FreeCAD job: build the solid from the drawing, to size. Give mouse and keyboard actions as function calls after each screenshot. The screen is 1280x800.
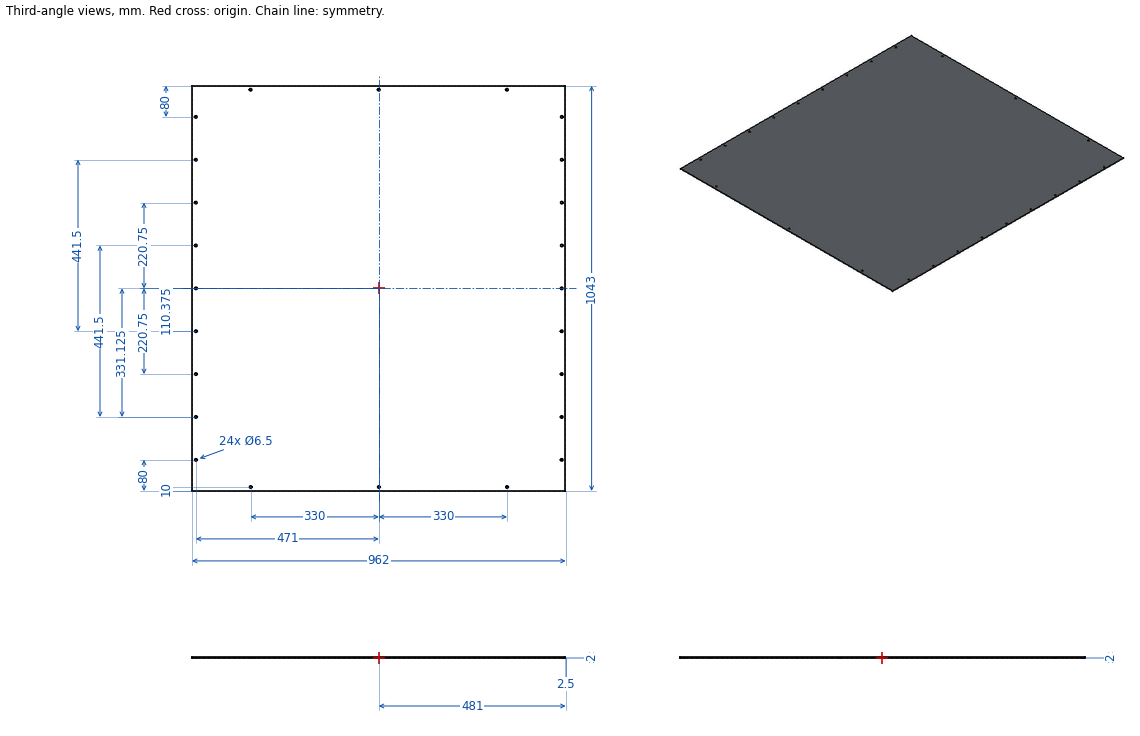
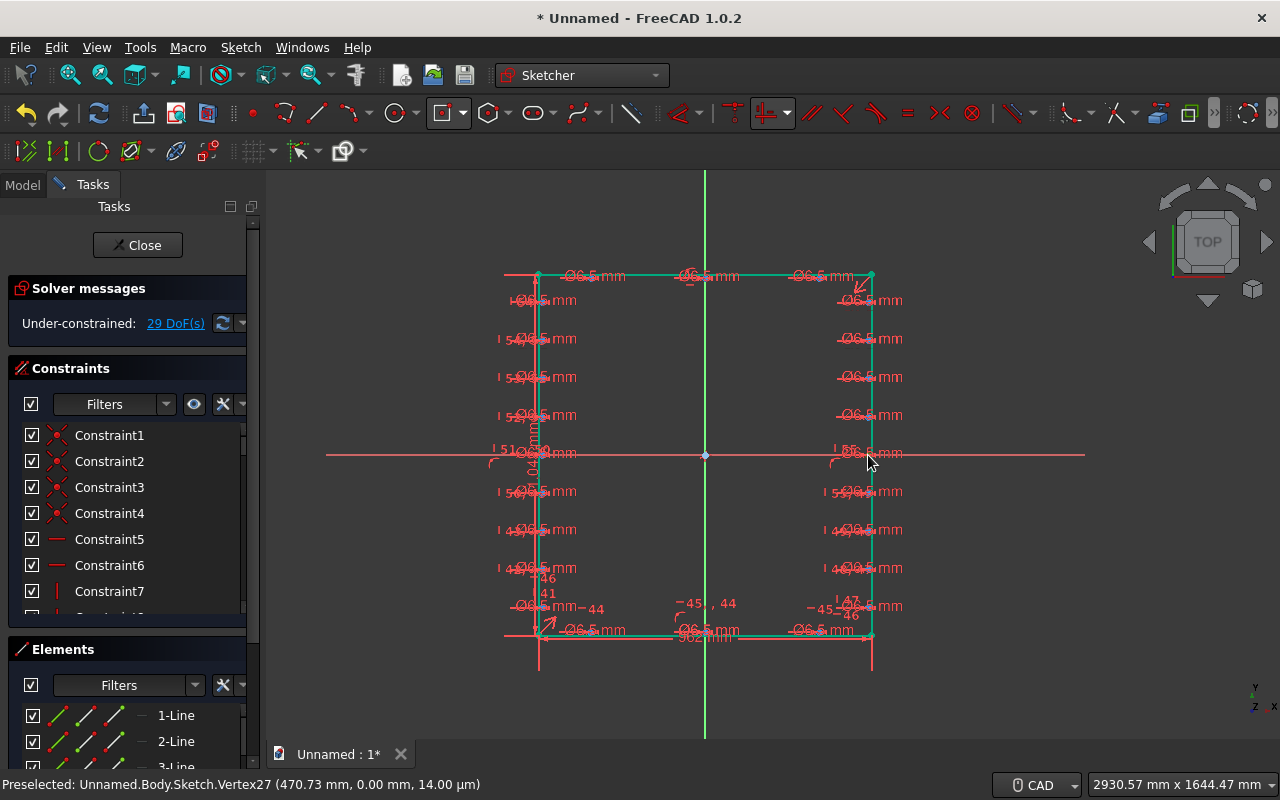
click(868, 417)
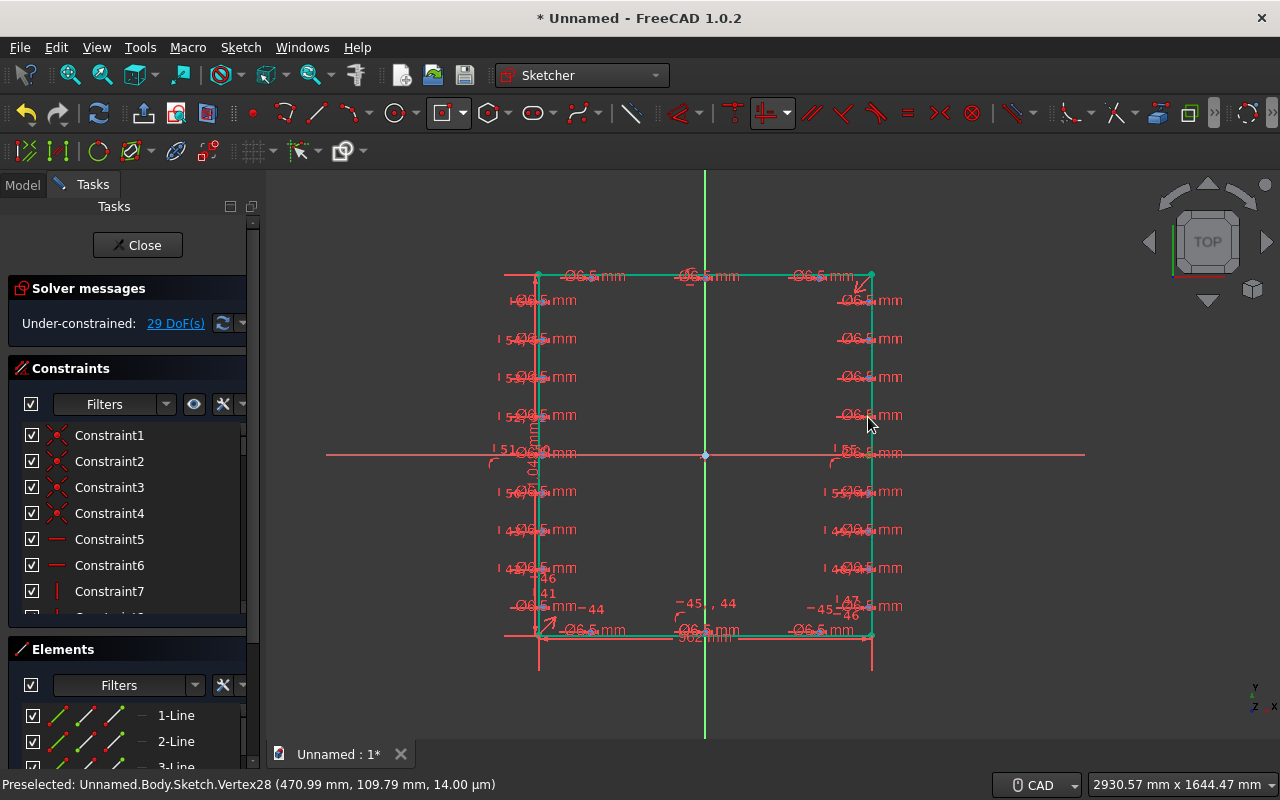
key(v)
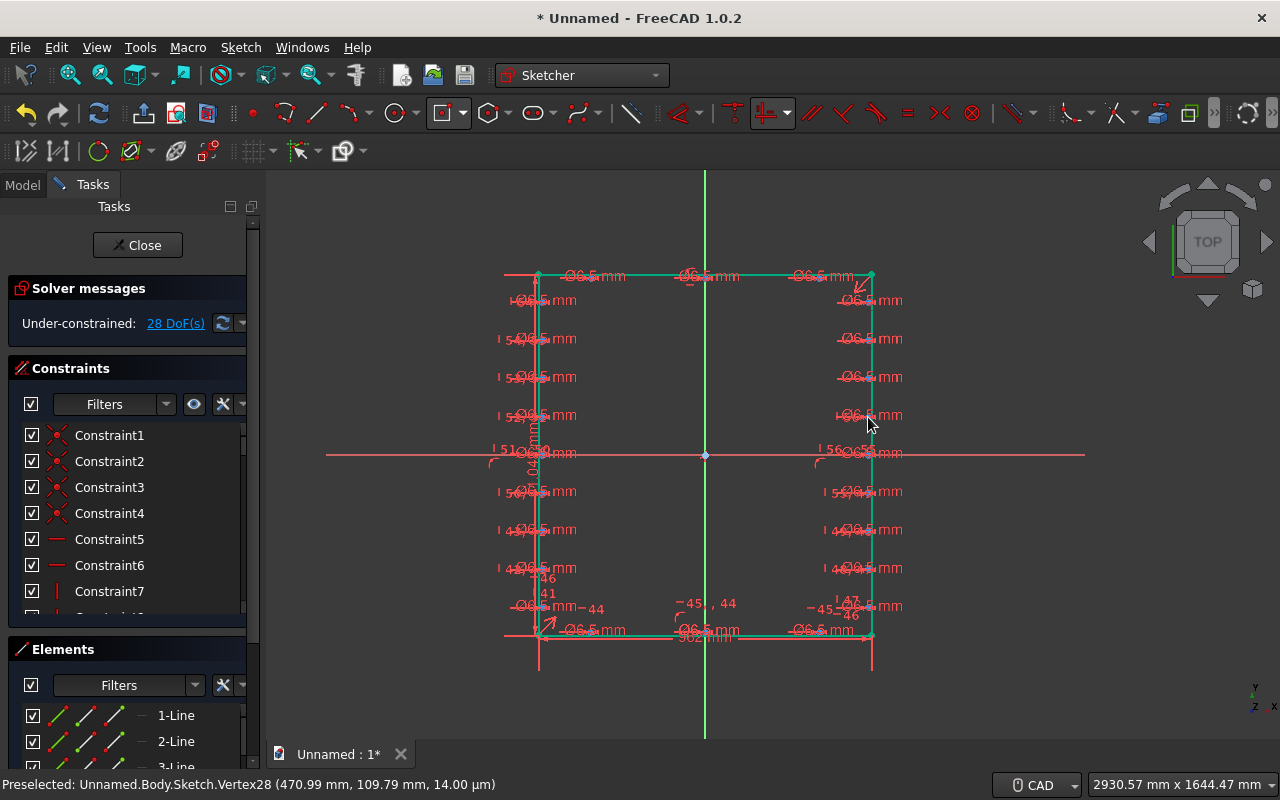
click(868, 417)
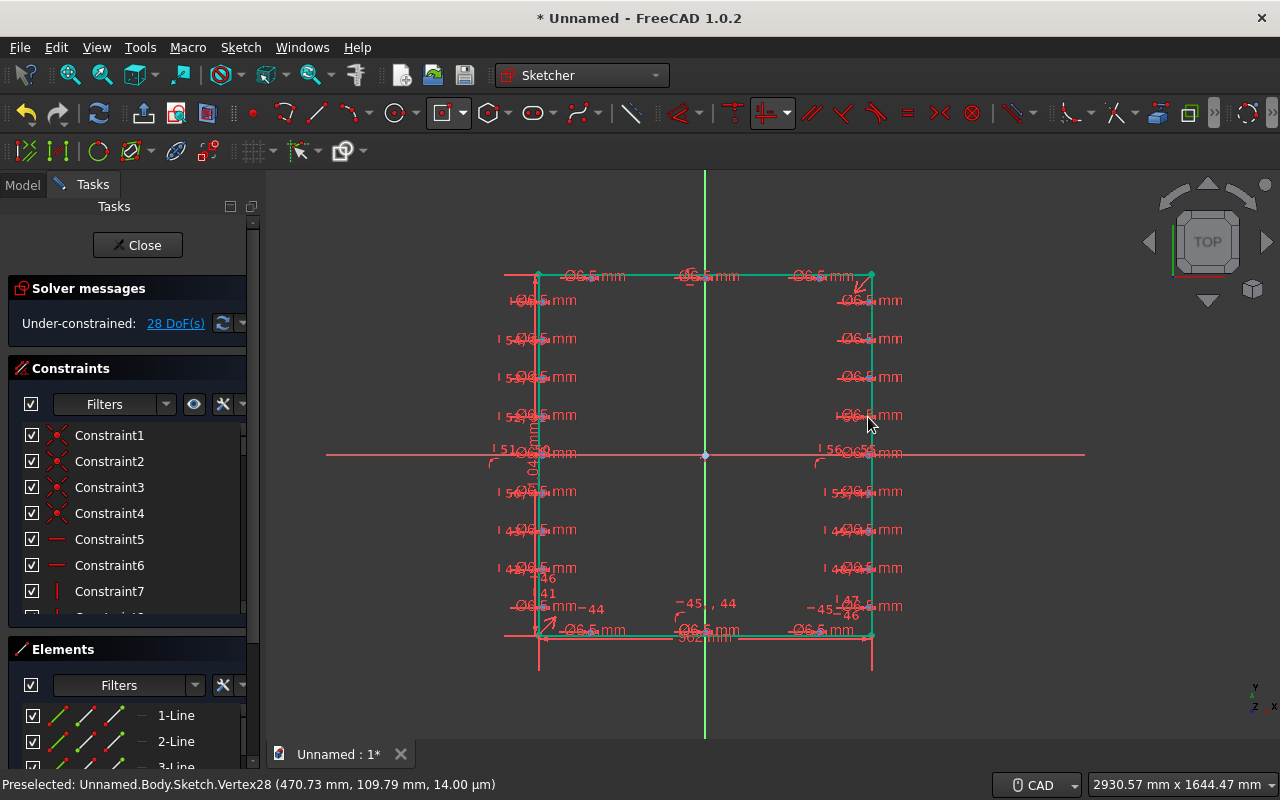
click(868, 379)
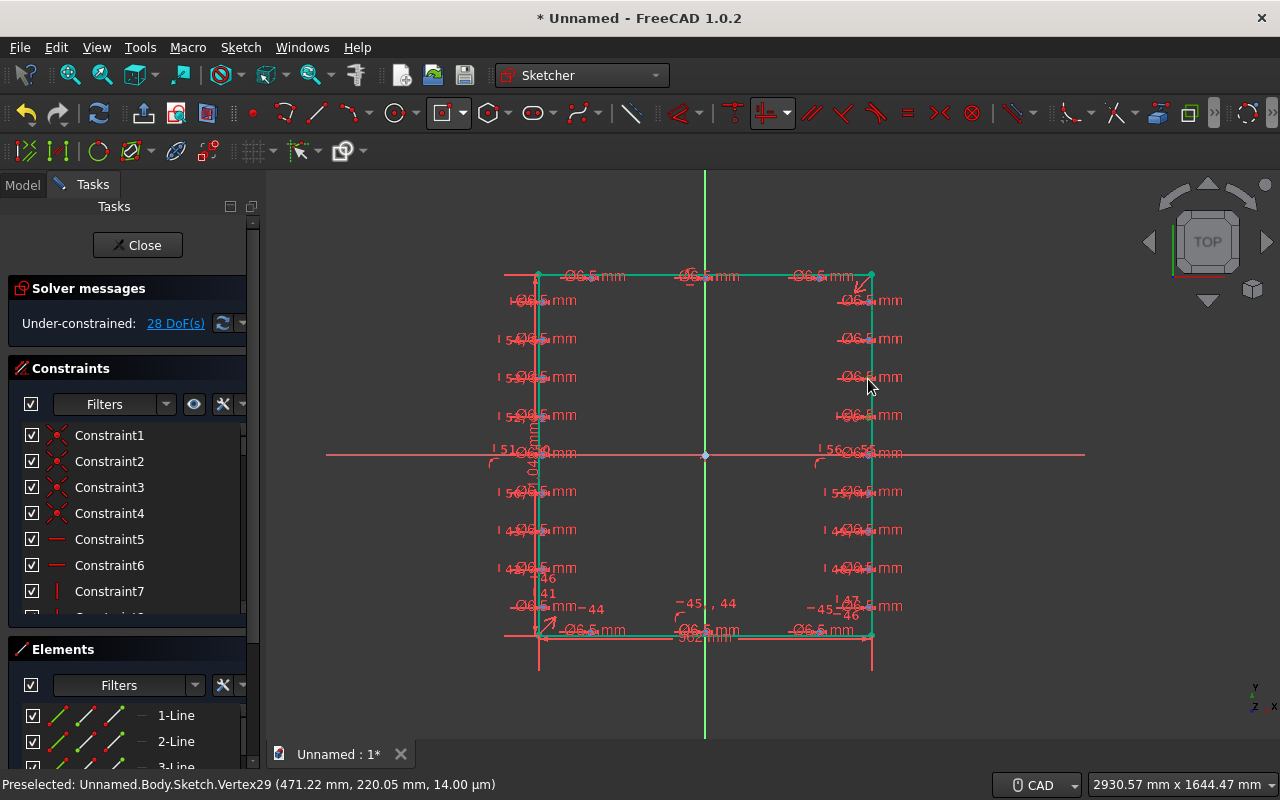
click(790, 114)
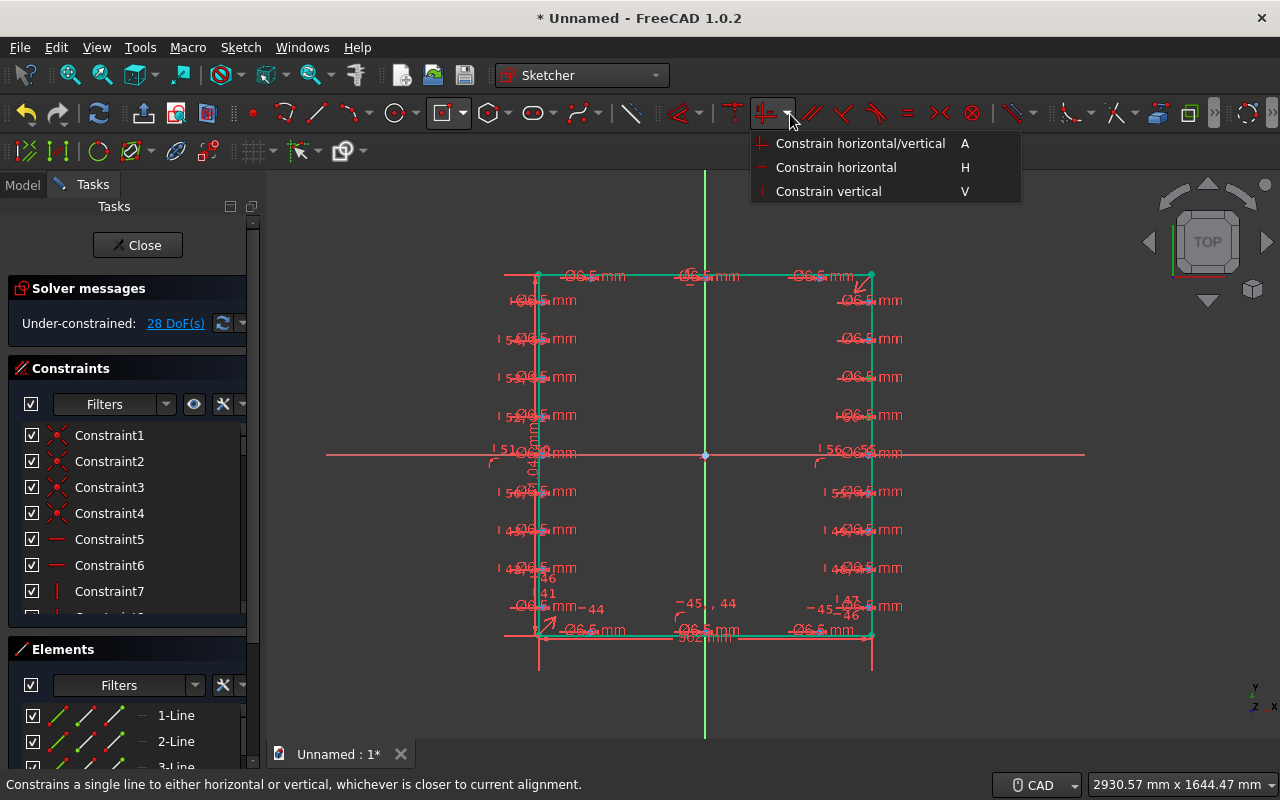
click(886, 191)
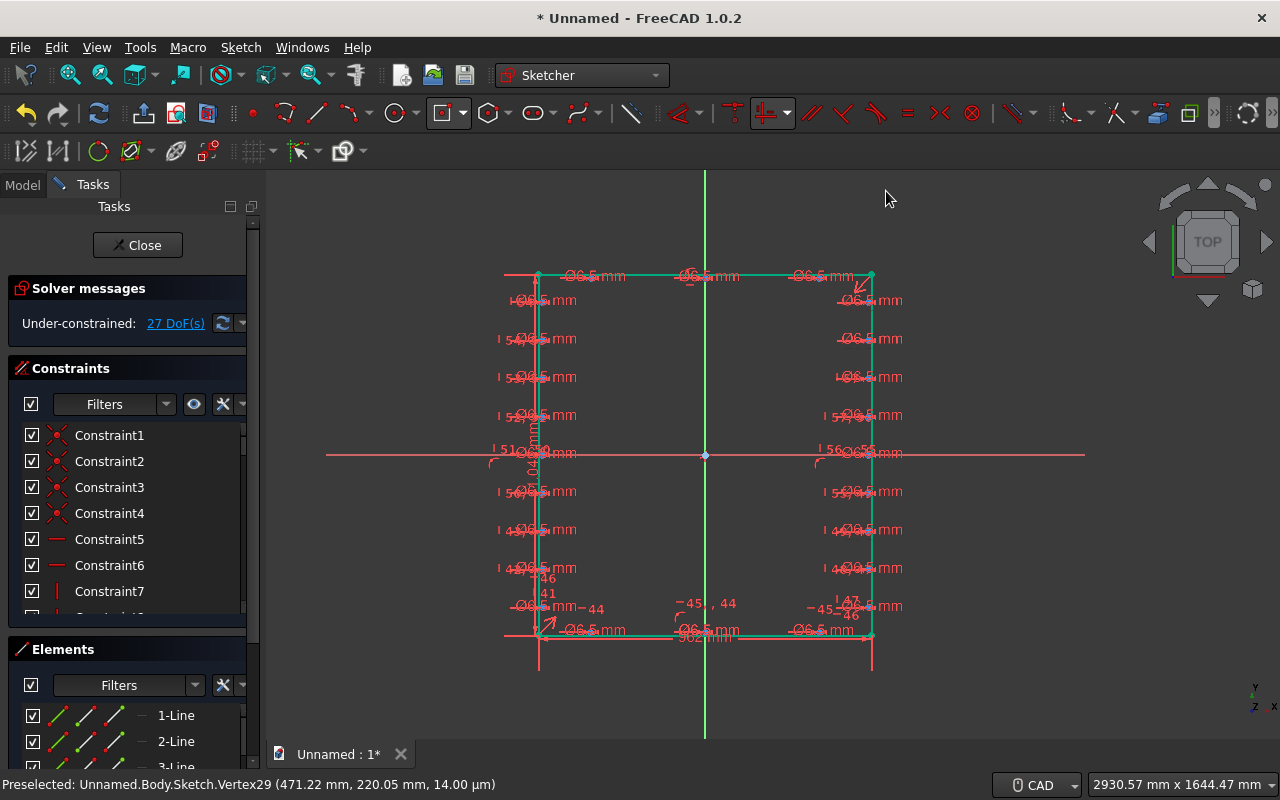
click(591, 278)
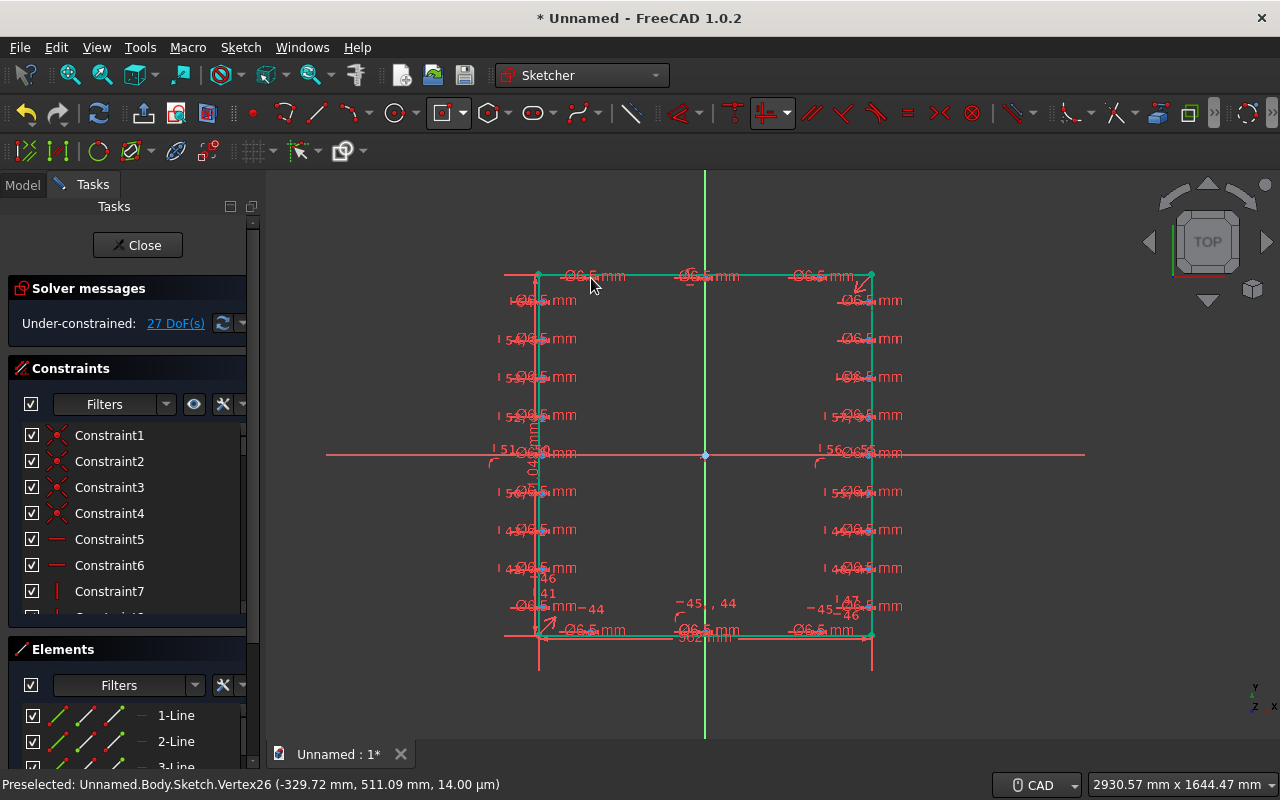
click(705, 278)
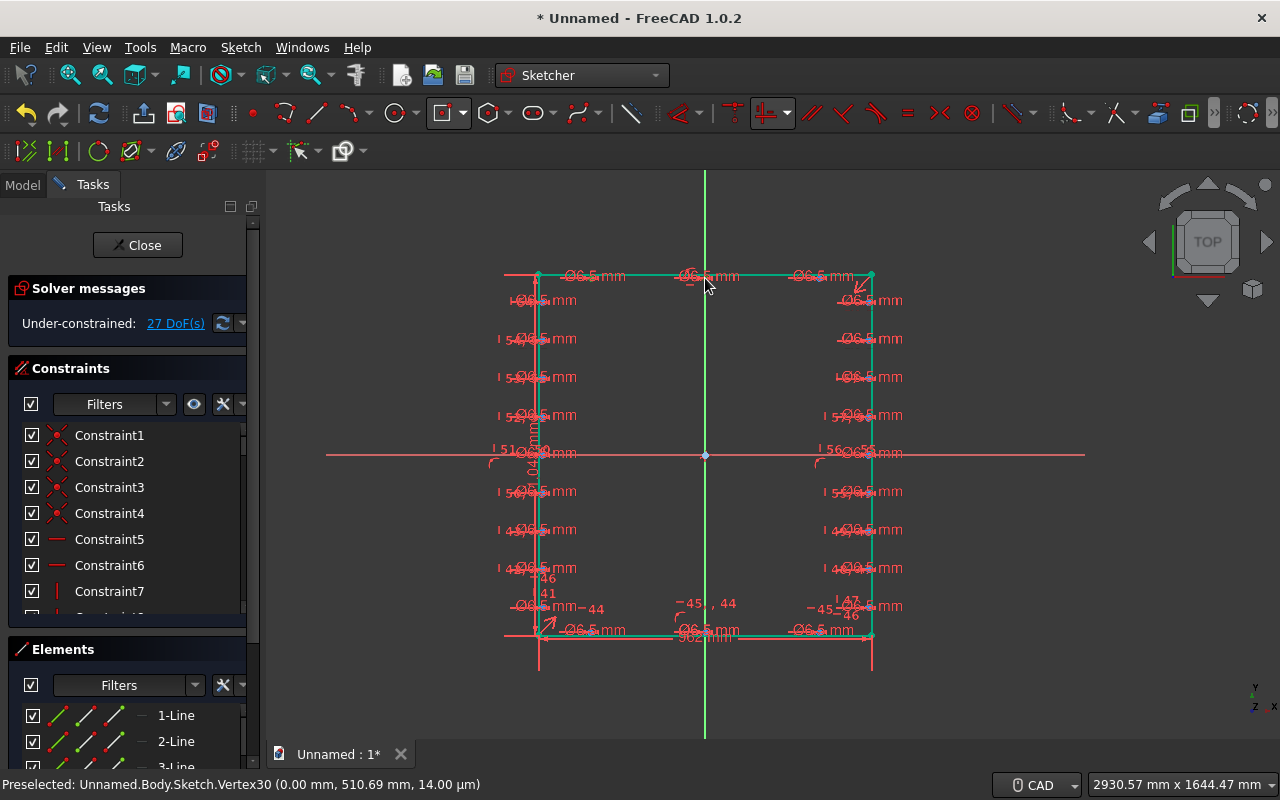
key(h)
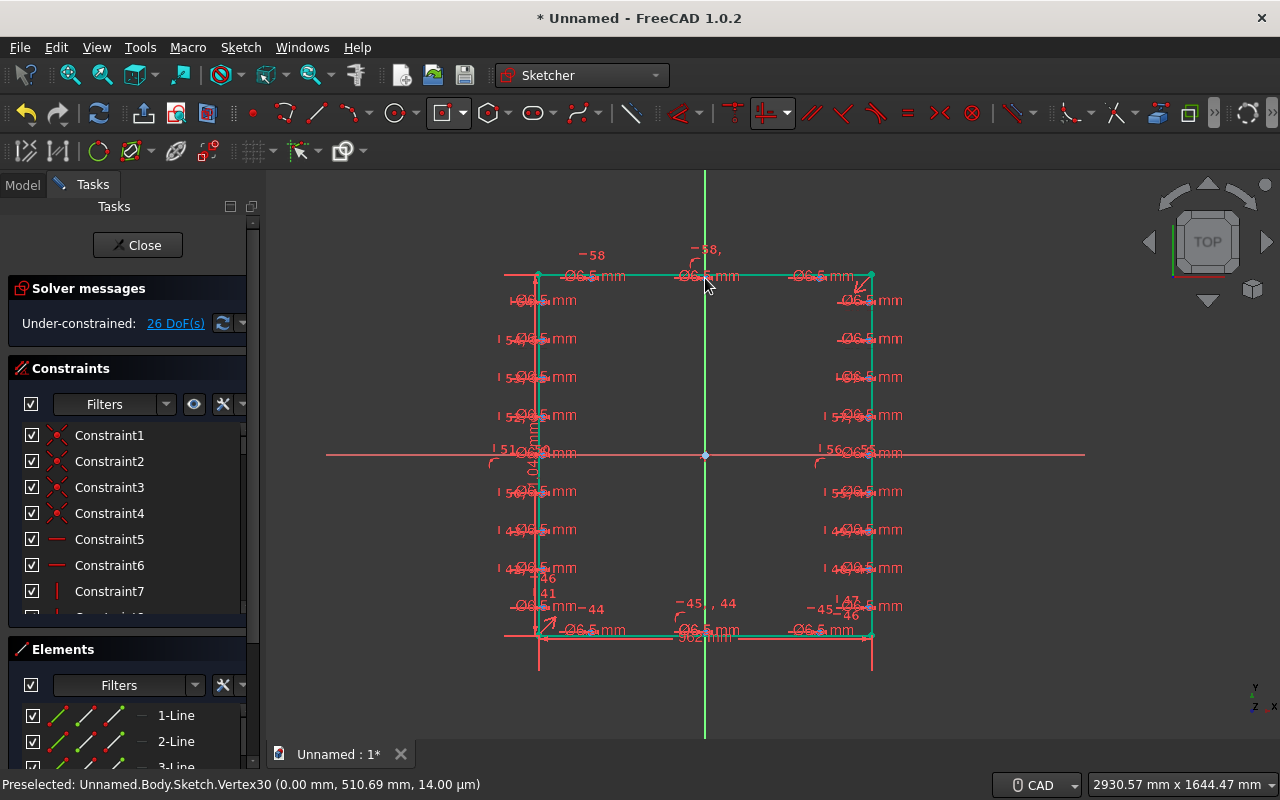
click(868, 379)